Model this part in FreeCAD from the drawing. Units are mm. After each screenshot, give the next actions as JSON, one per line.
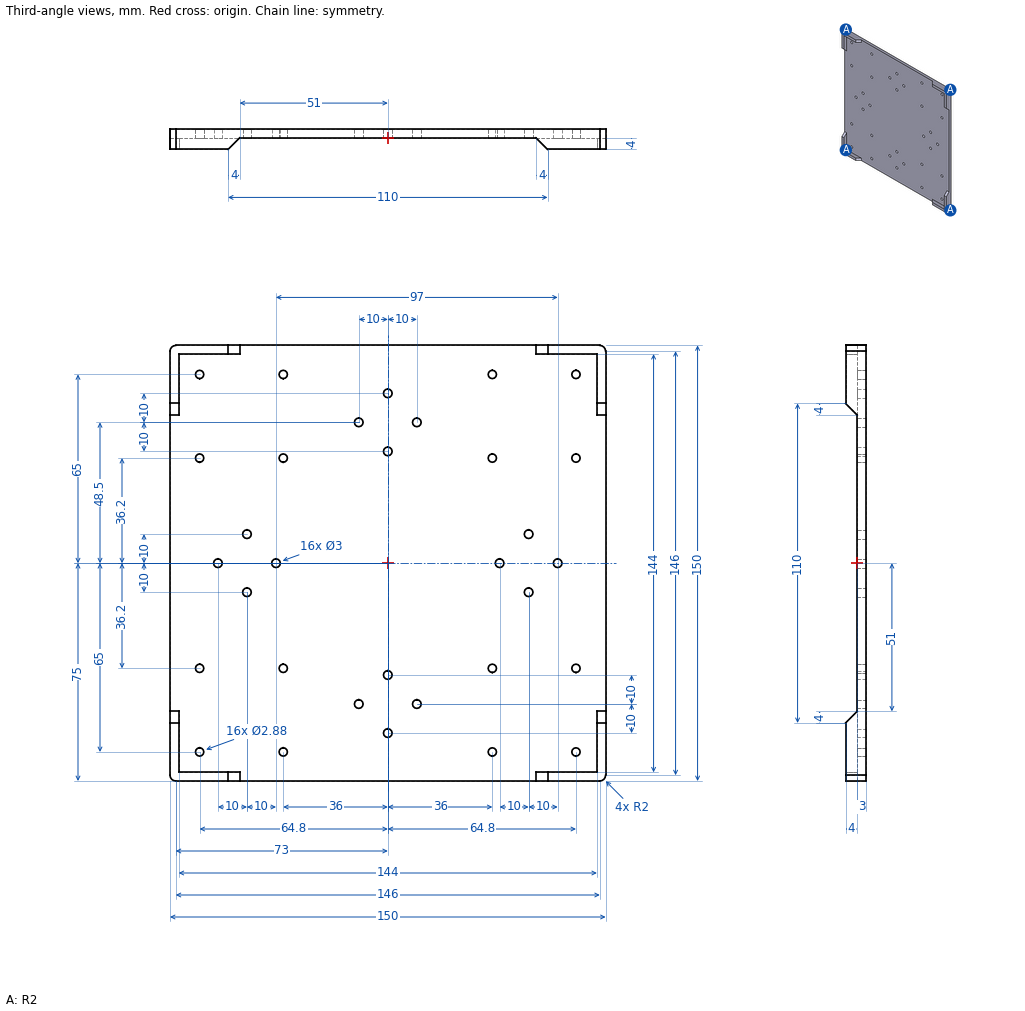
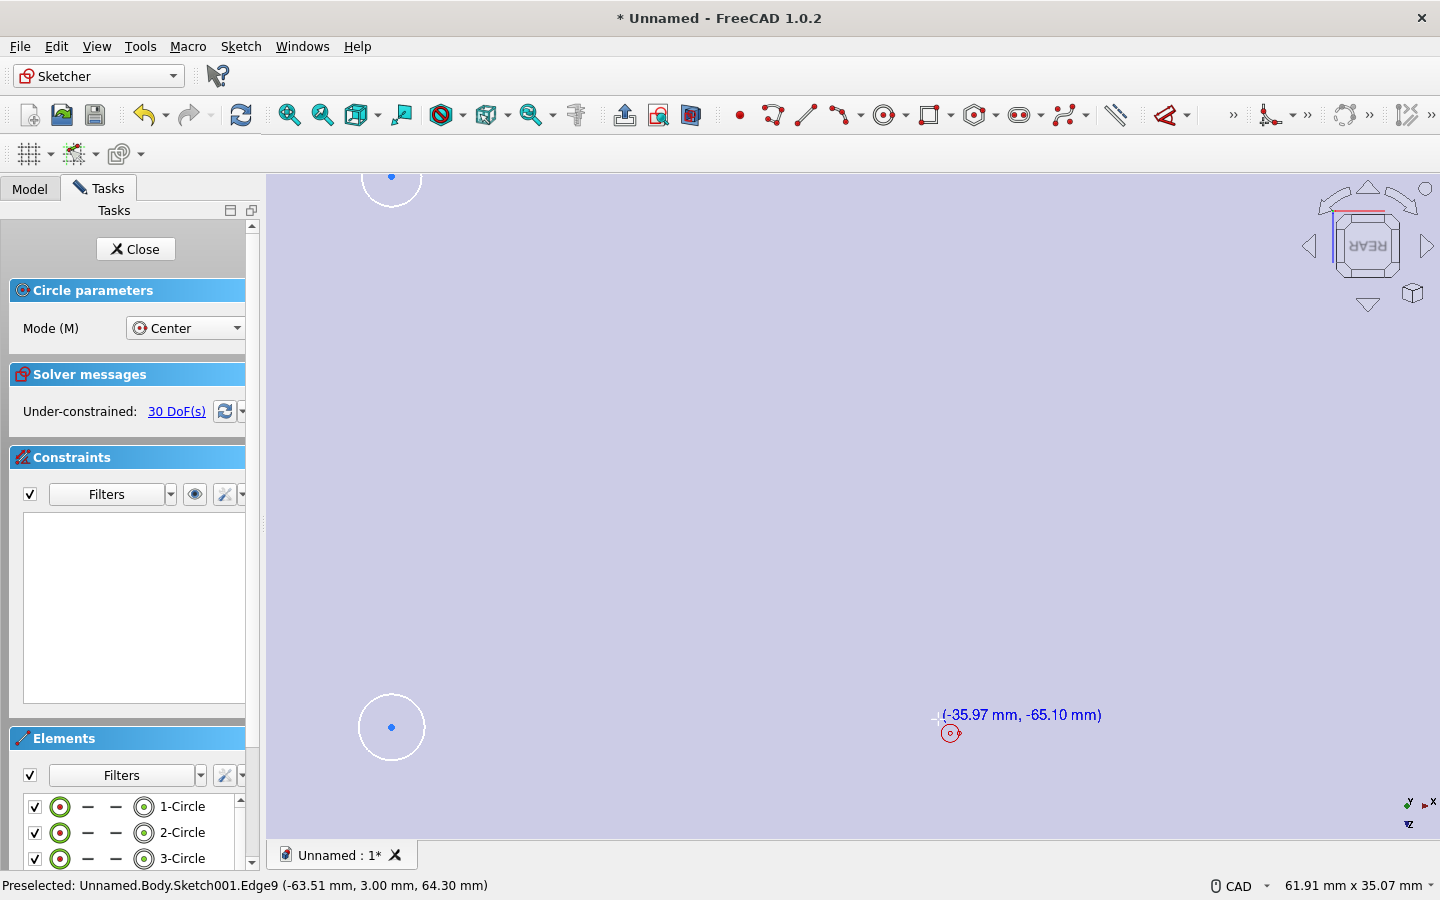
{"action": "scroll", "coordinate": [619, 709], "scroll_direction": "down", "scroll_amount": 9}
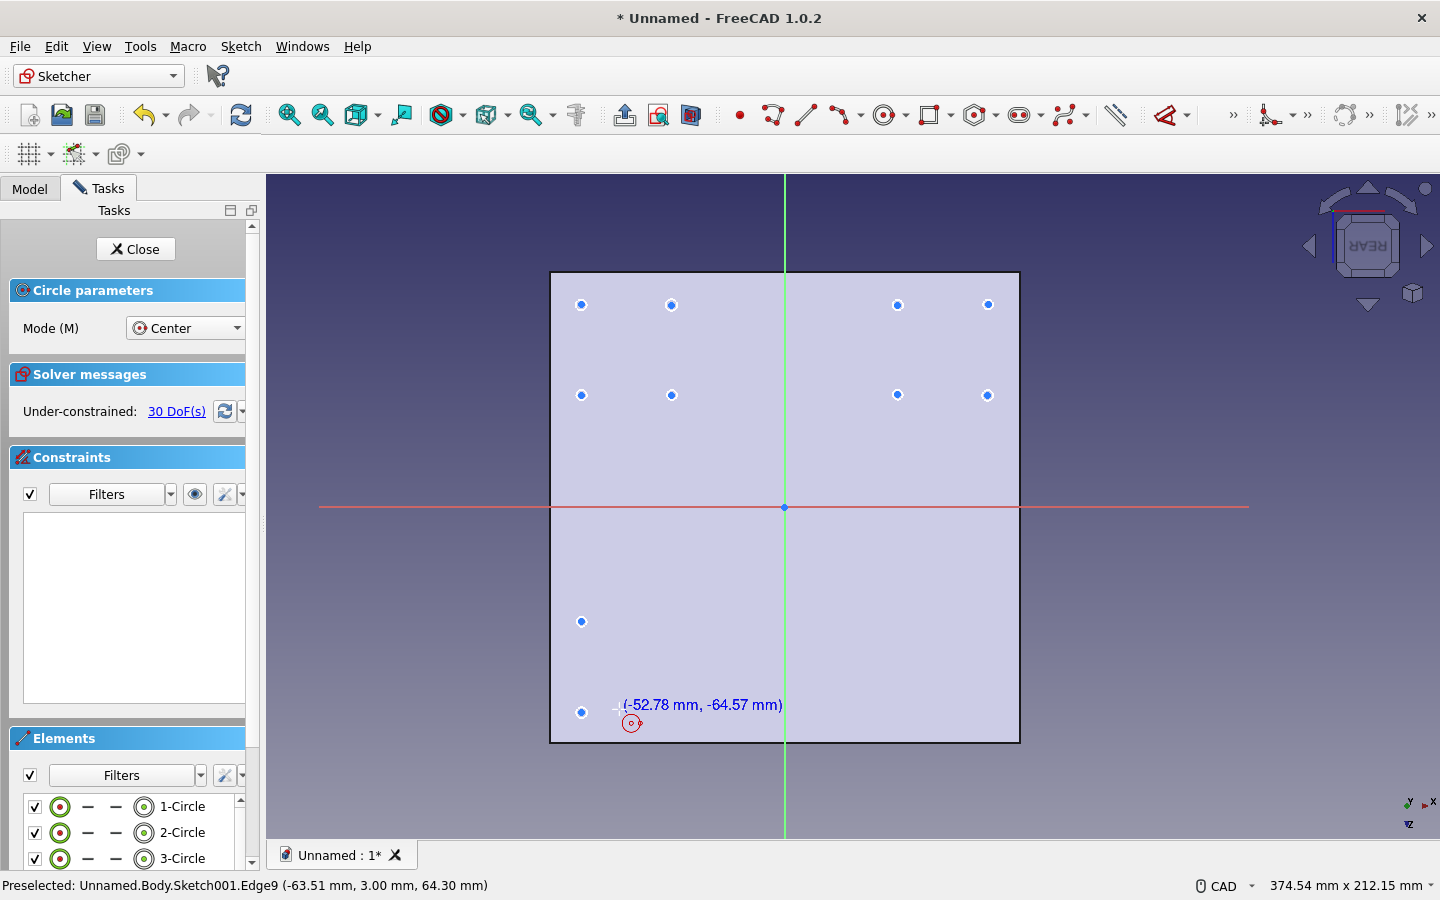
{"action": "left_click", "coordinate": [672, 711]}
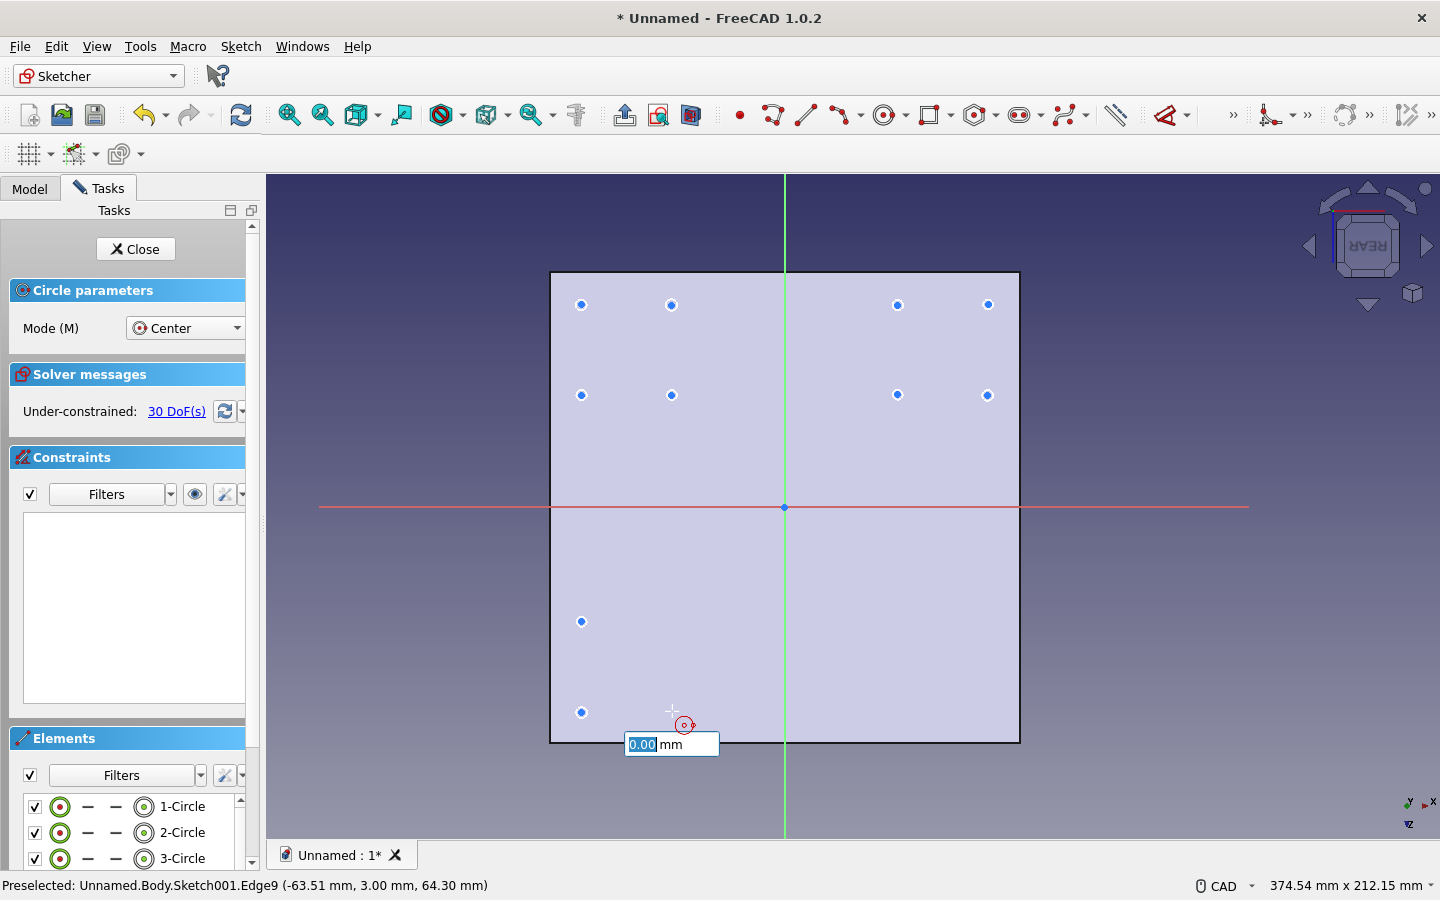
{"action": "scroll", "coordinate": [675, 708], "scroll_direction": "up", "scroll_amount": 7}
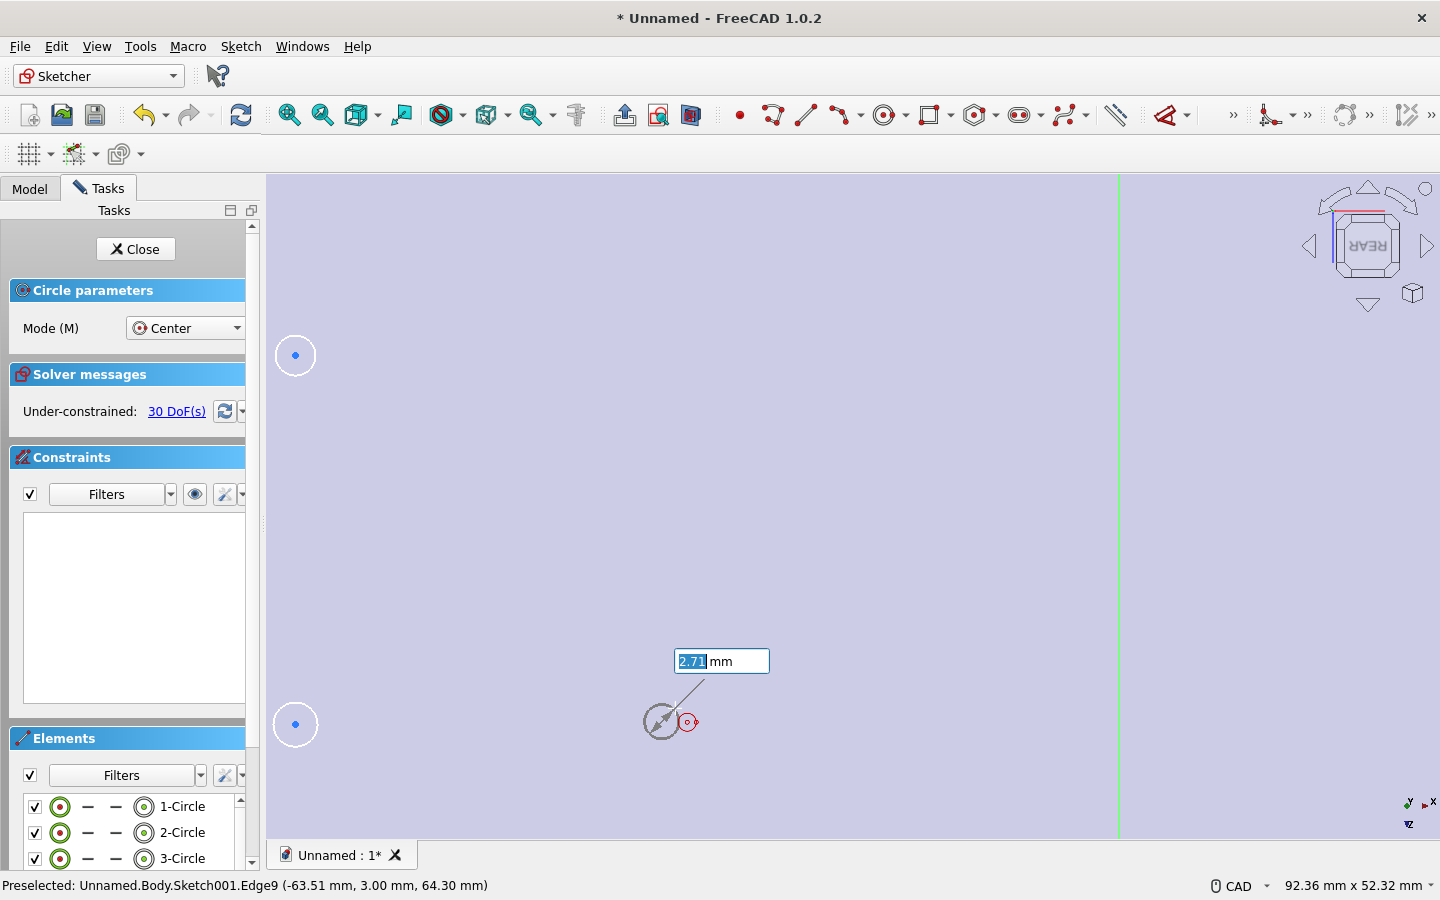
{"action": "left_click", "coordinate": [674, 706]}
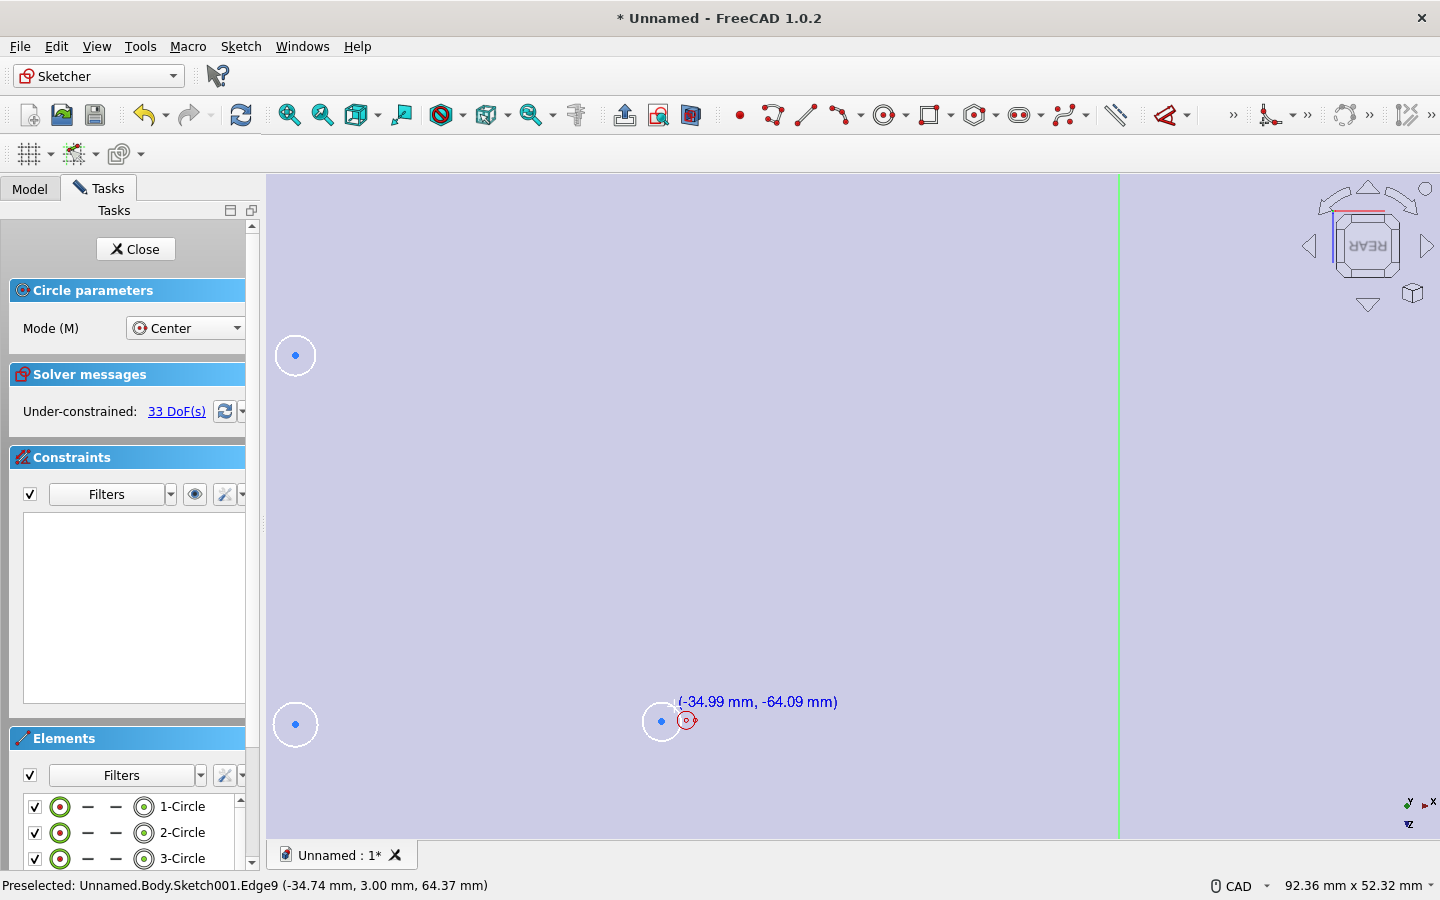
{"action": "scroll", "coordinate": [661, 352], "scroll_direction": "up", "scroll_amount": 2}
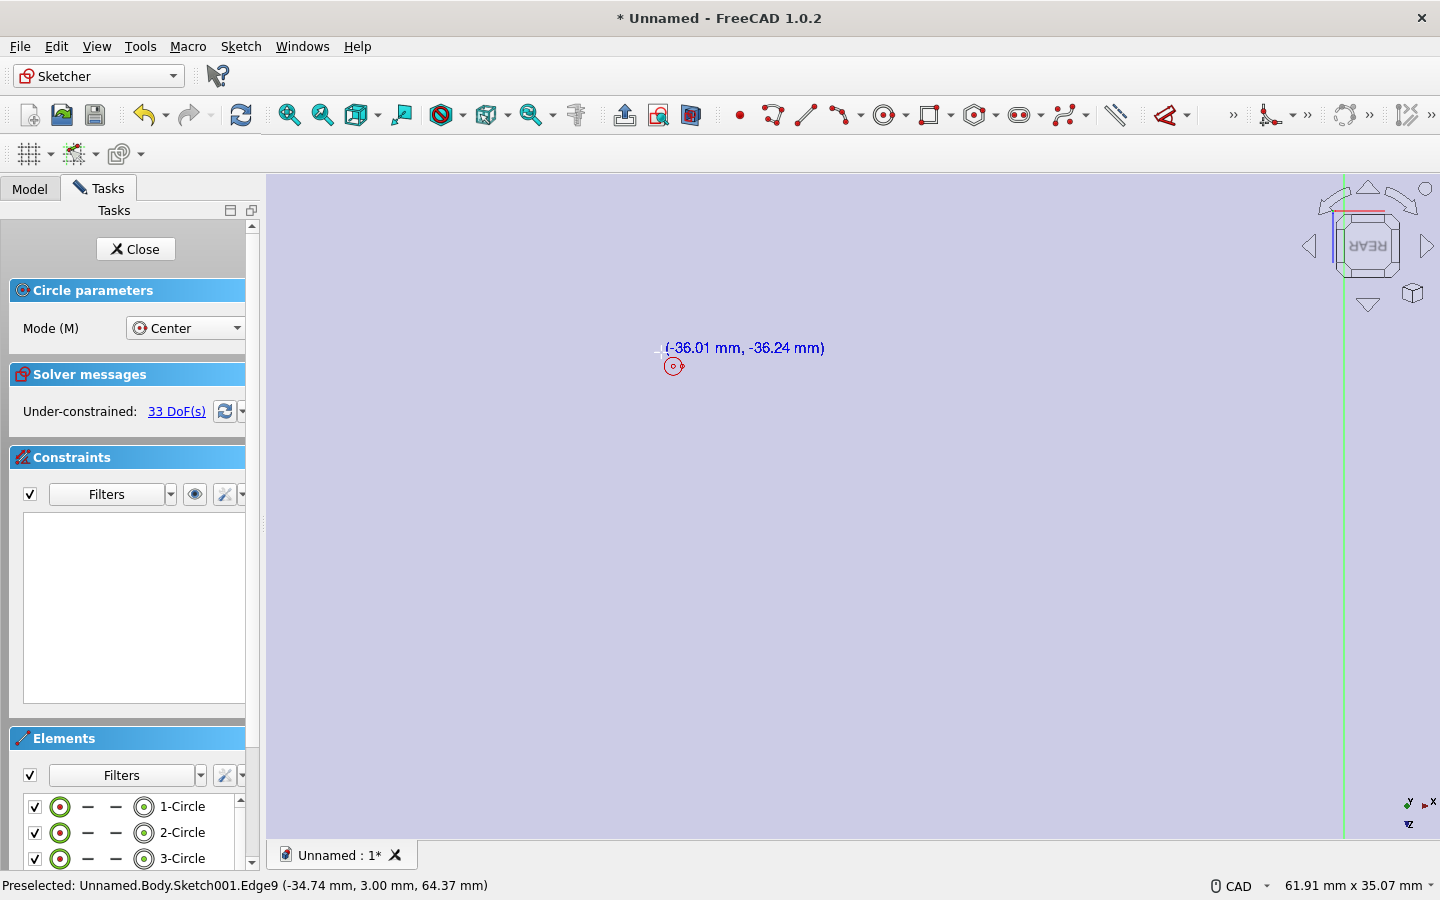
{"action": "scroll", "coordinate": [674, 673], "scroll_direction": "down", "scroll_amount": 9}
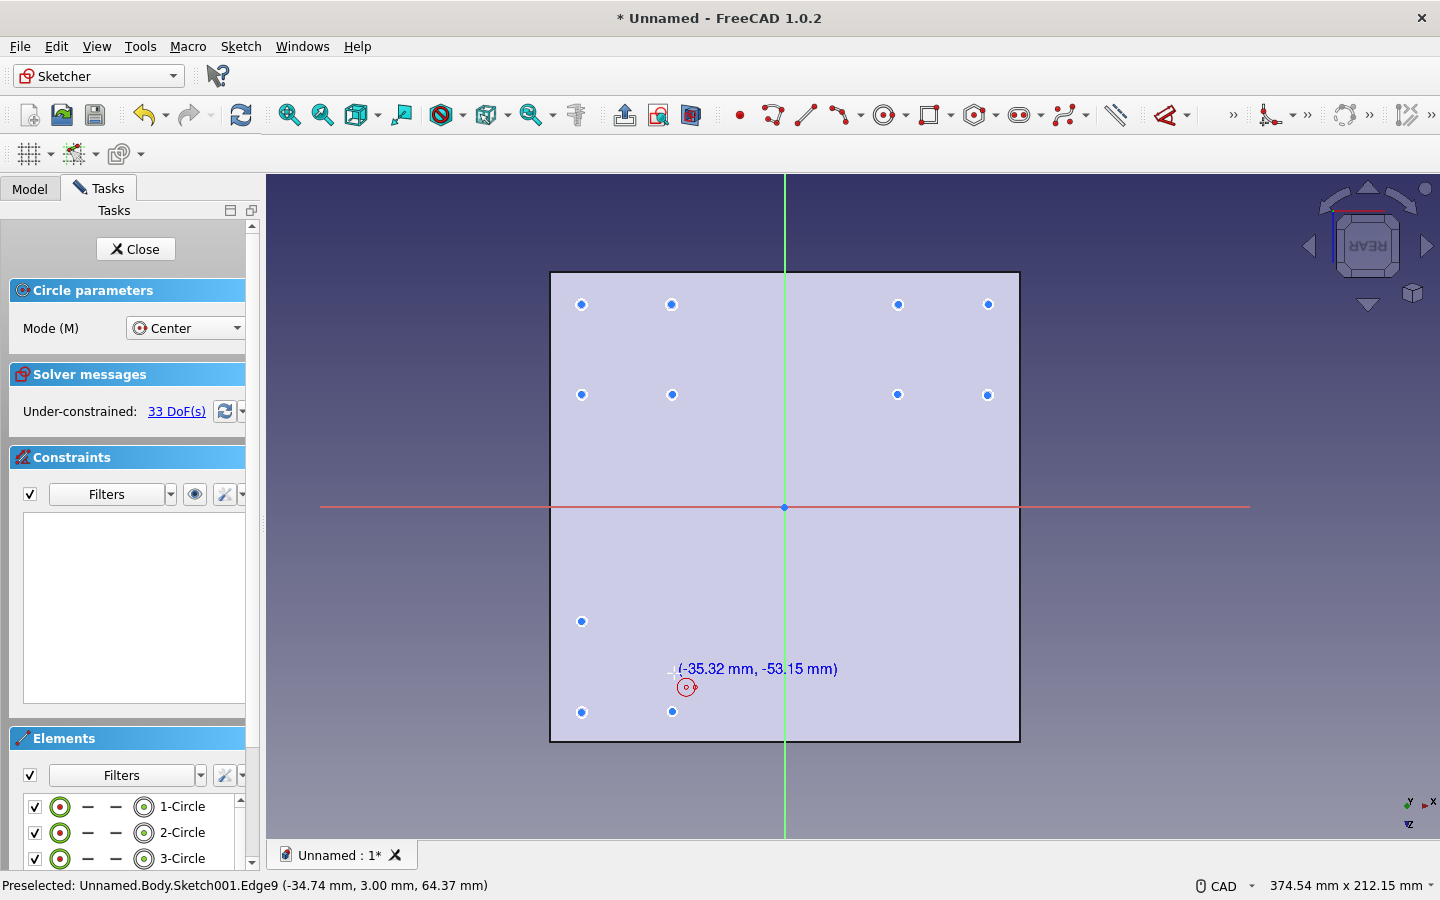
{"action": "left_click", "coordinate": [672, 621]}